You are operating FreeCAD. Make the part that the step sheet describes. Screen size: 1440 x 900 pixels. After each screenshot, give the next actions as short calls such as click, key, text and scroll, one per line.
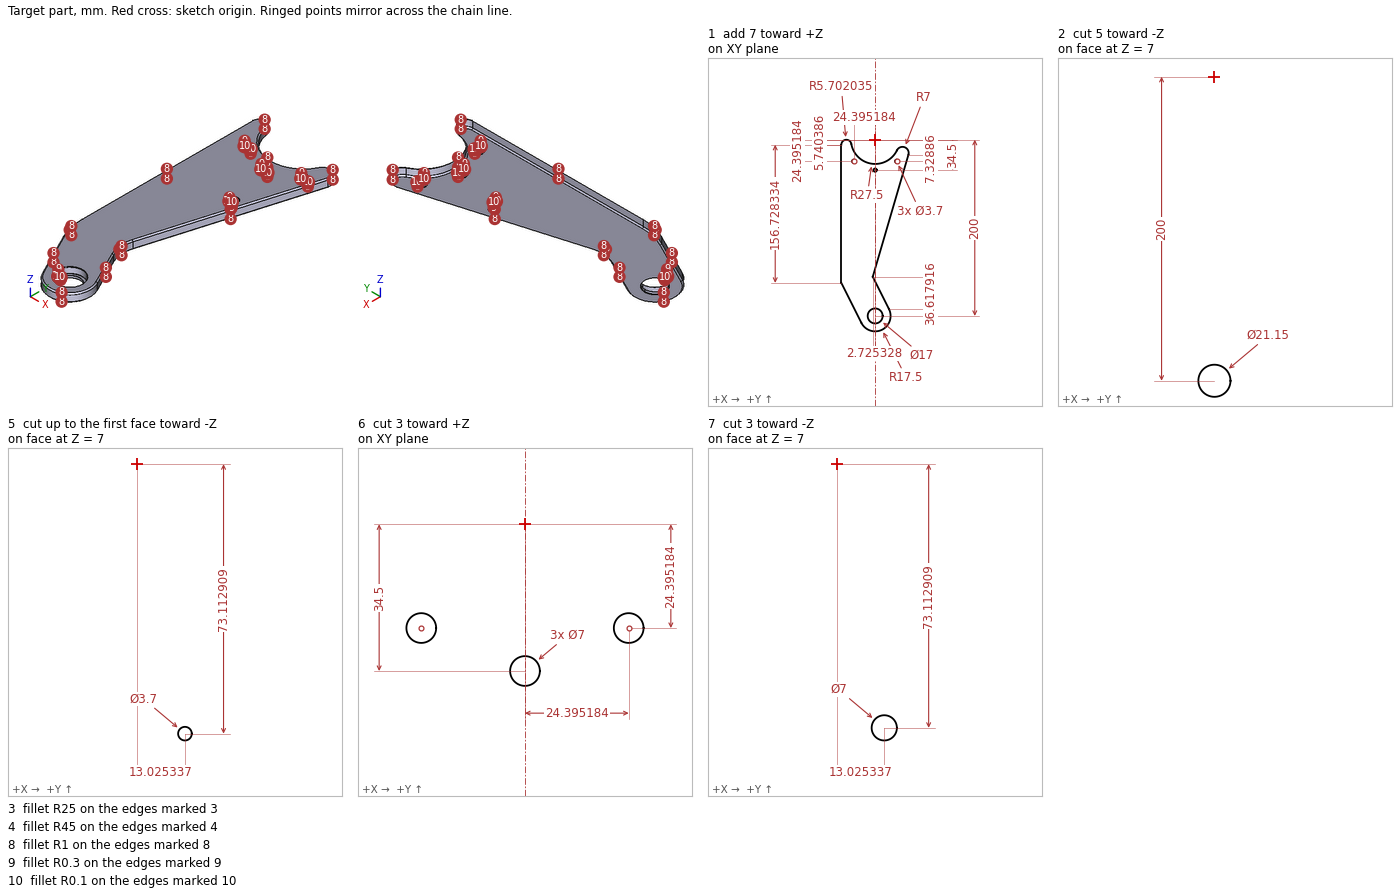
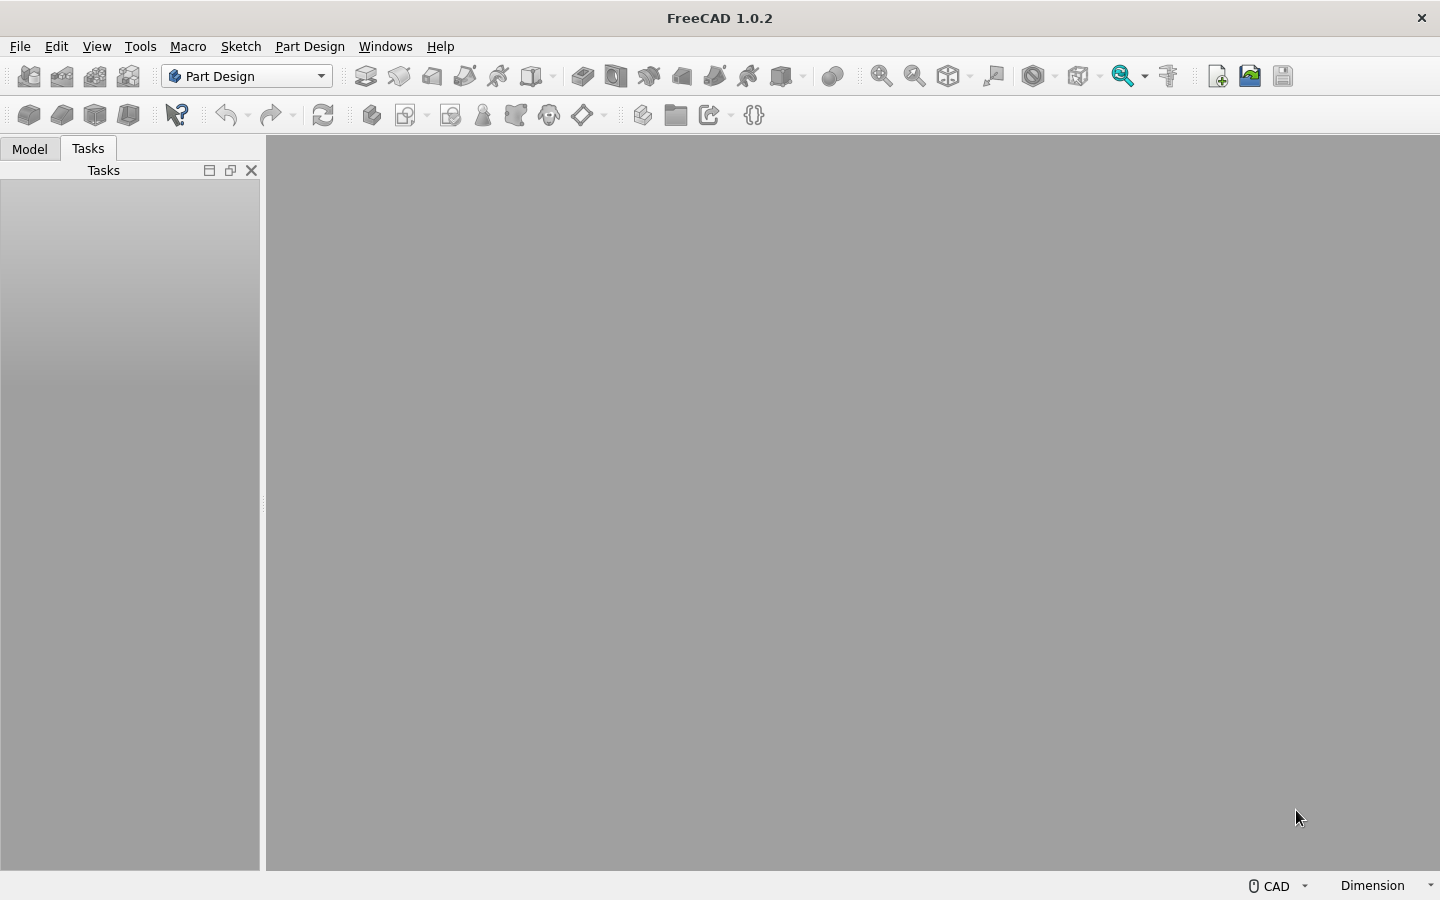
click(1217, 76)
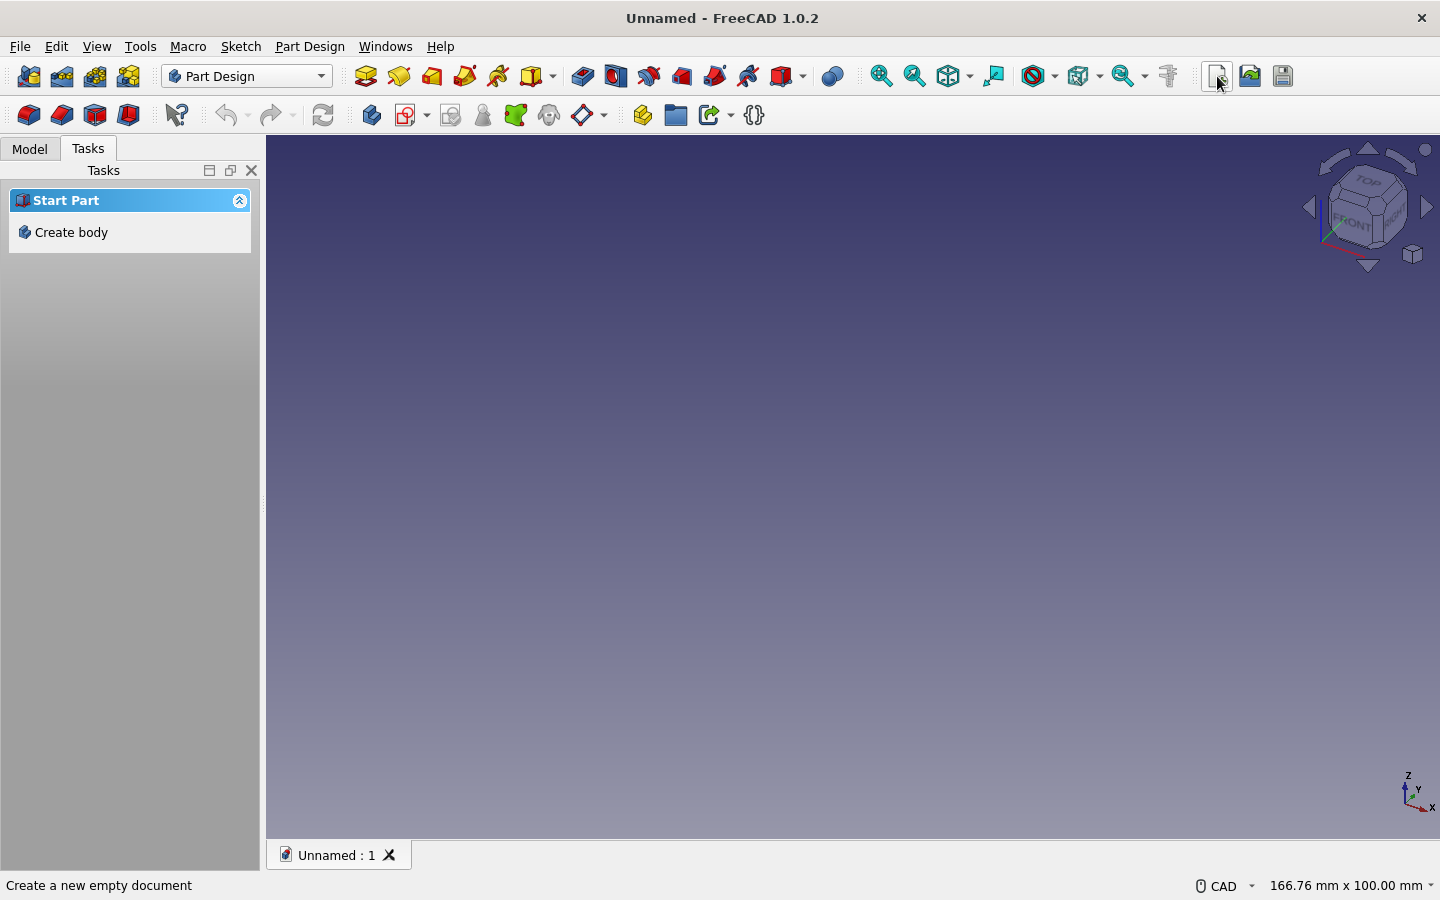
click(404, 116)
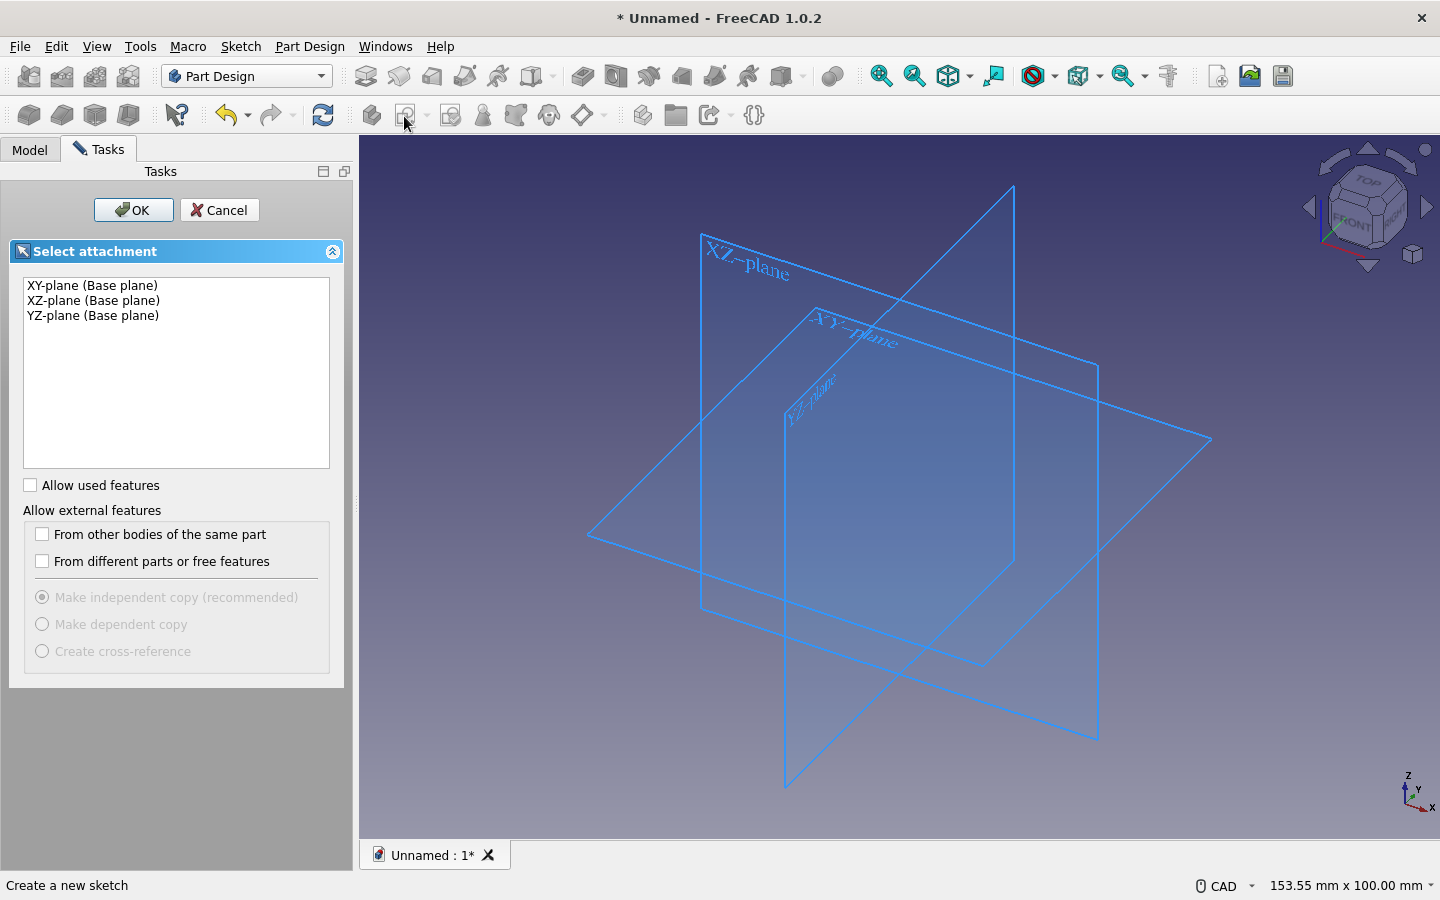
click(84, 286)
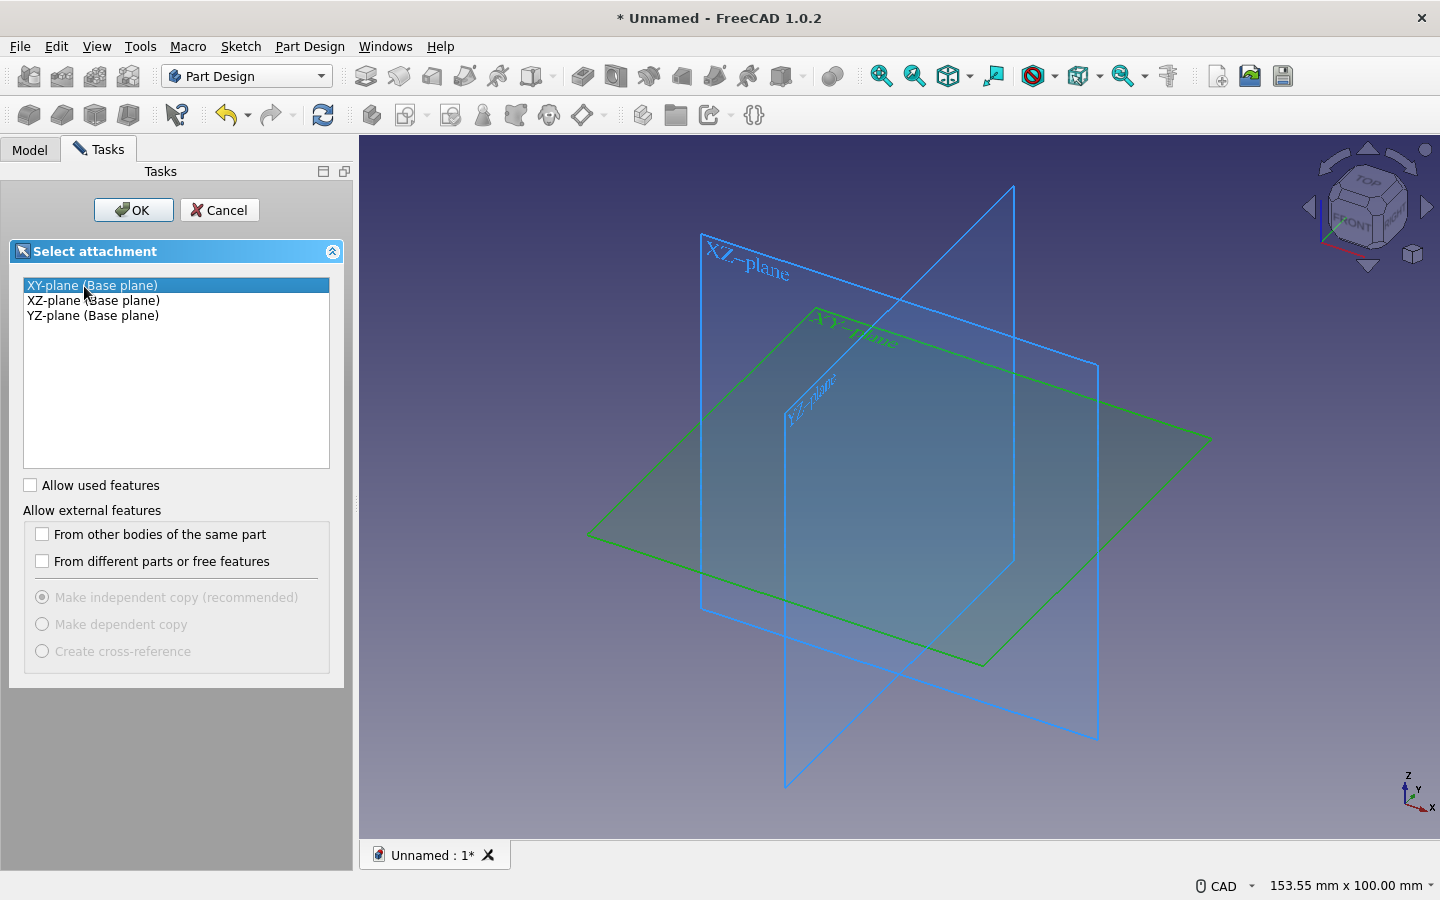
click(134, 210)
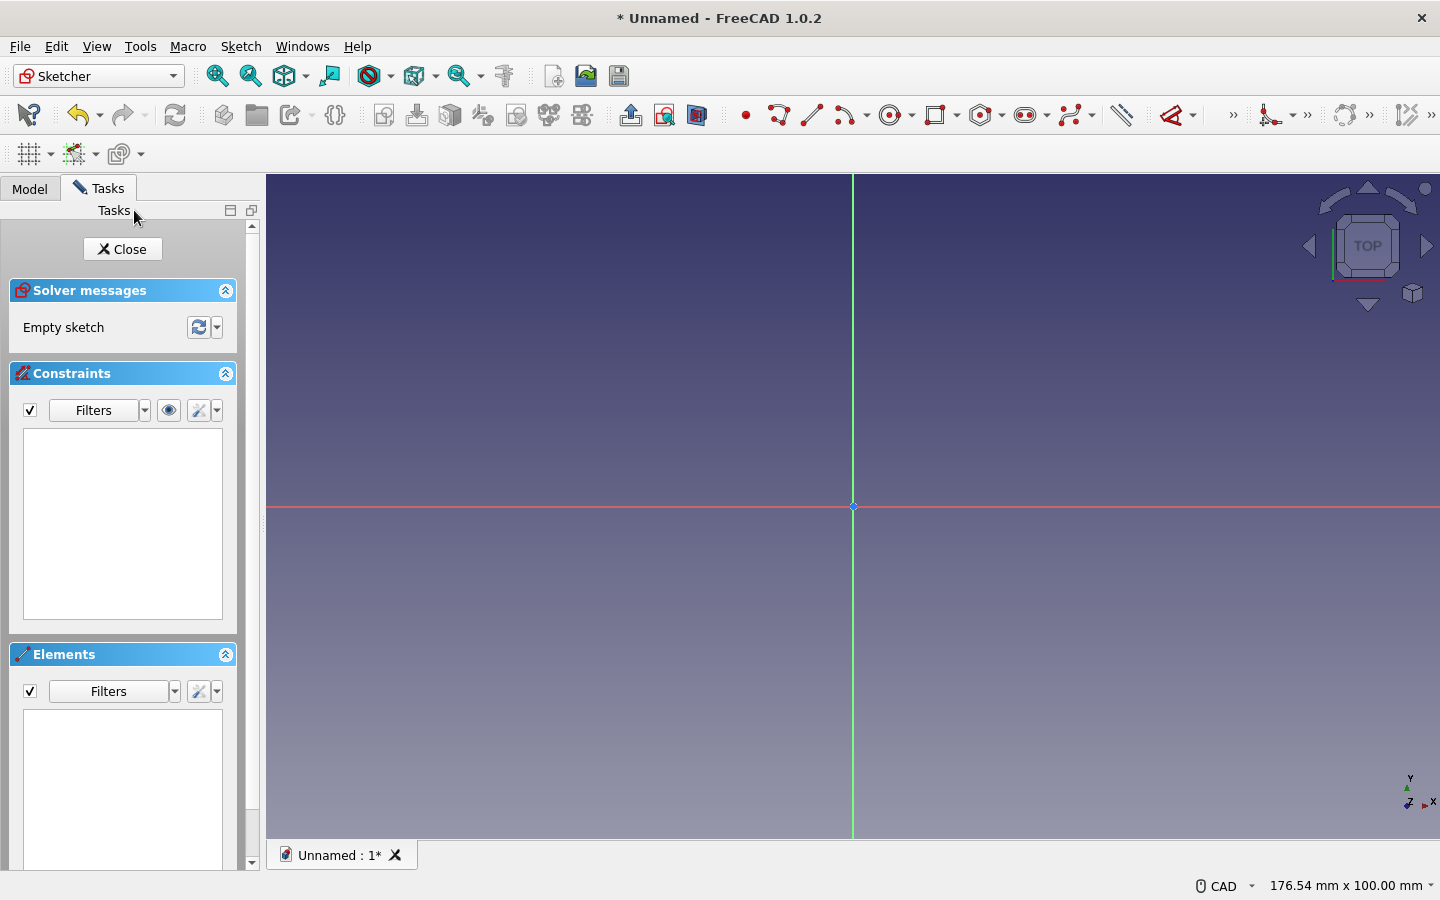
scroll(756, 202, down, 6)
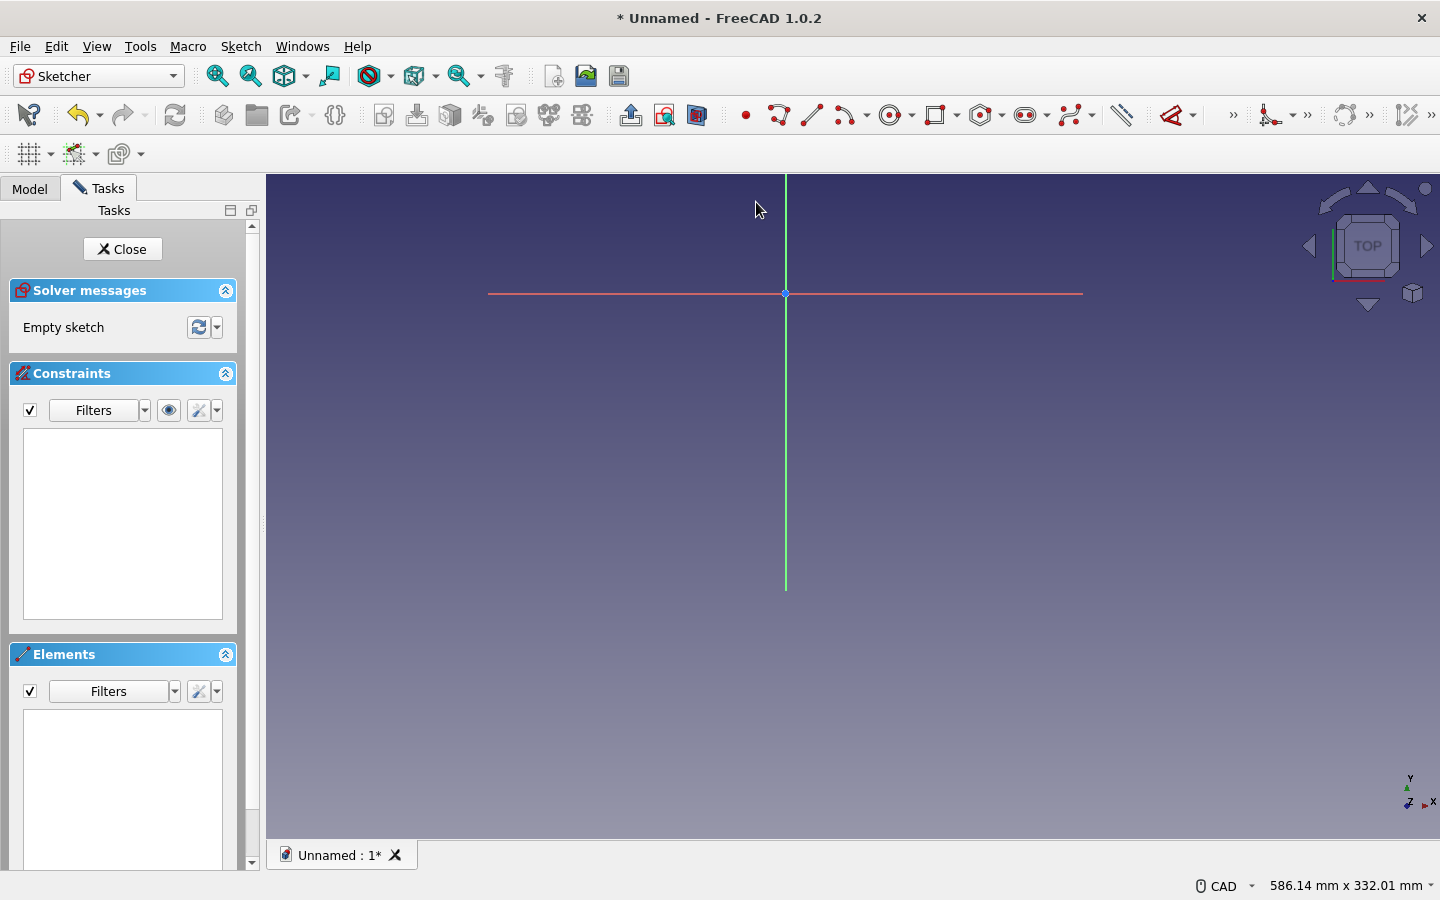
click(779, 116)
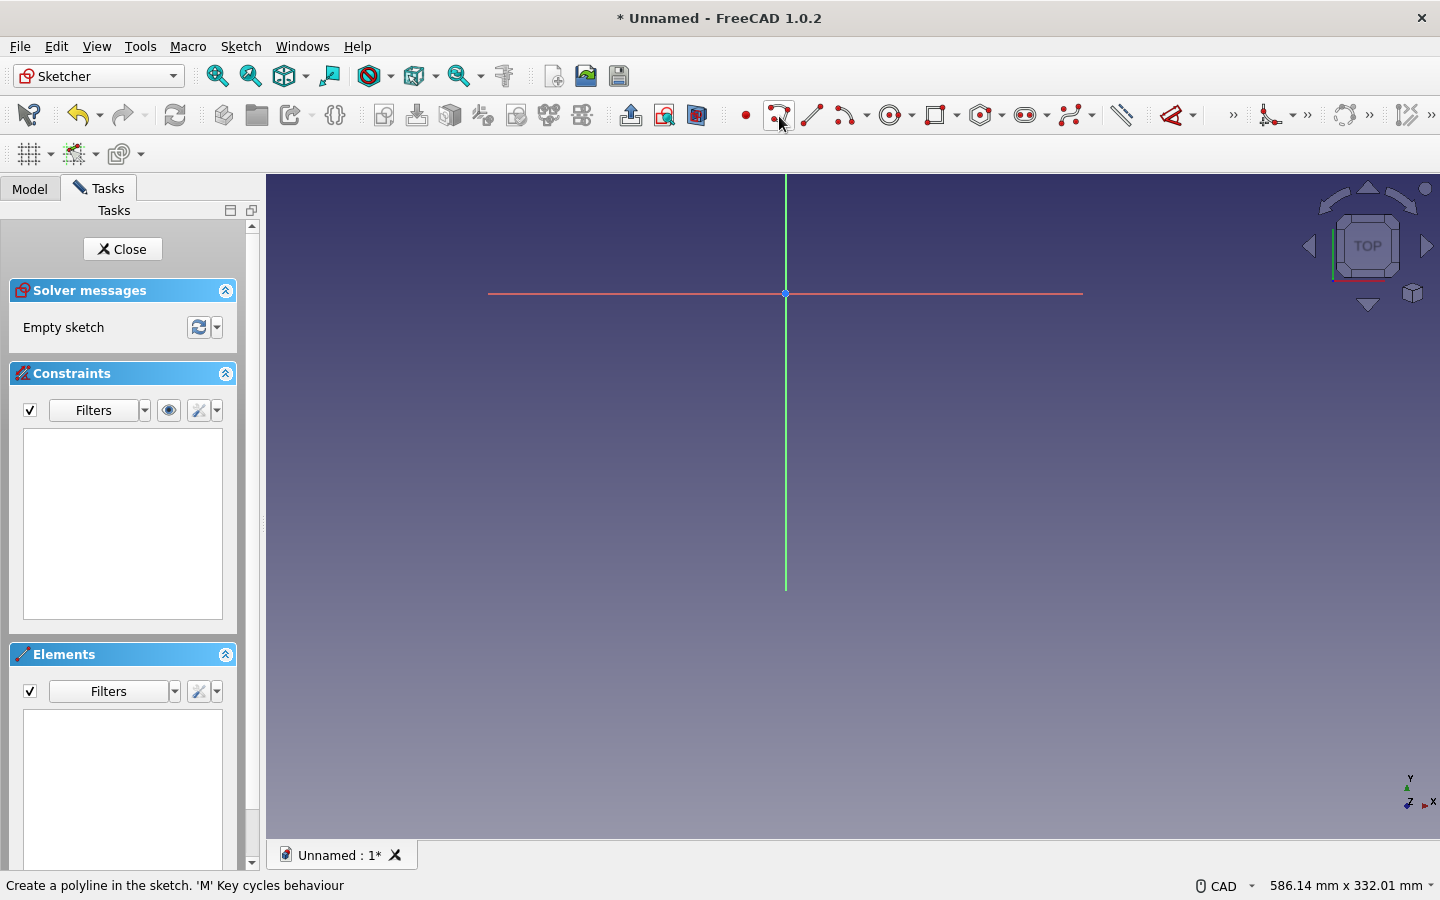
scroll(709, 305, up, 2)